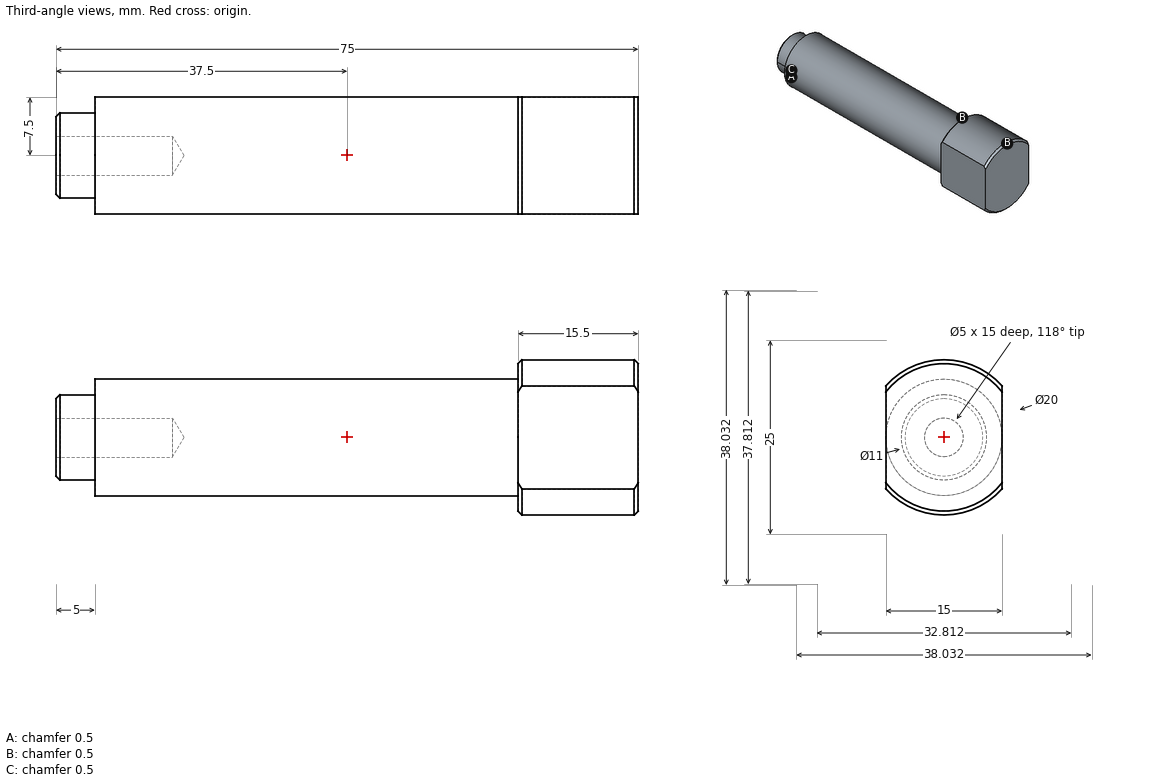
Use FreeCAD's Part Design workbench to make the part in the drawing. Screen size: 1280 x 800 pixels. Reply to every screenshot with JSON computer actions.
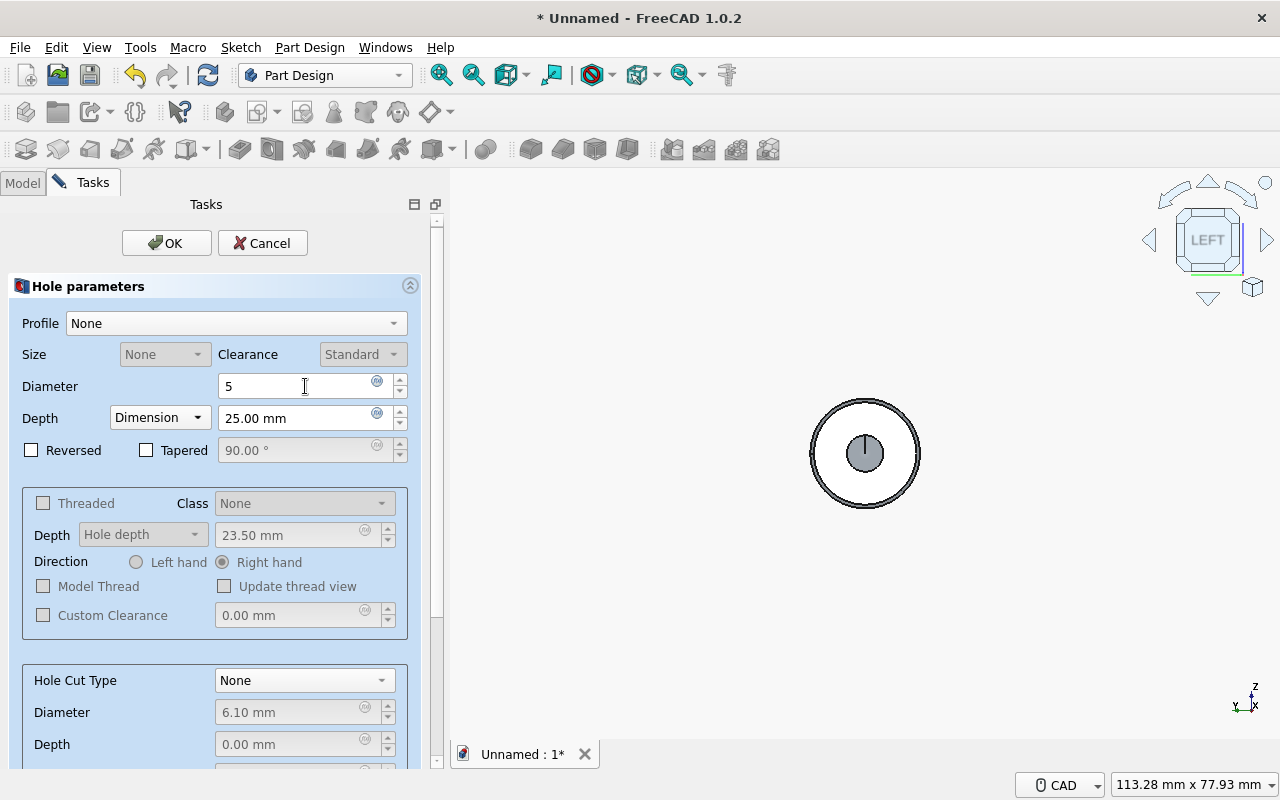
{"action": "triple_click", "coordinate": [305, 418]}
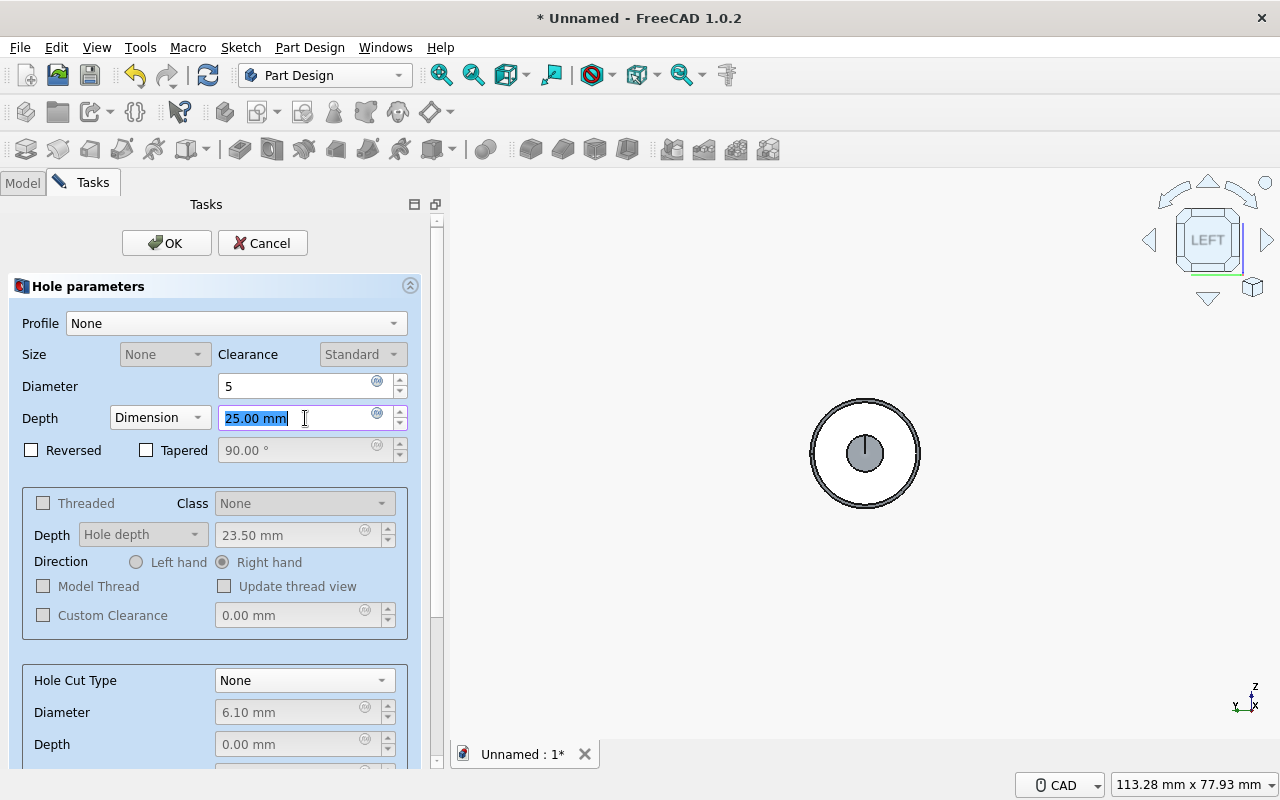
{"action": "type", "text": "15"}
{"action": "key", "text": "Tab"}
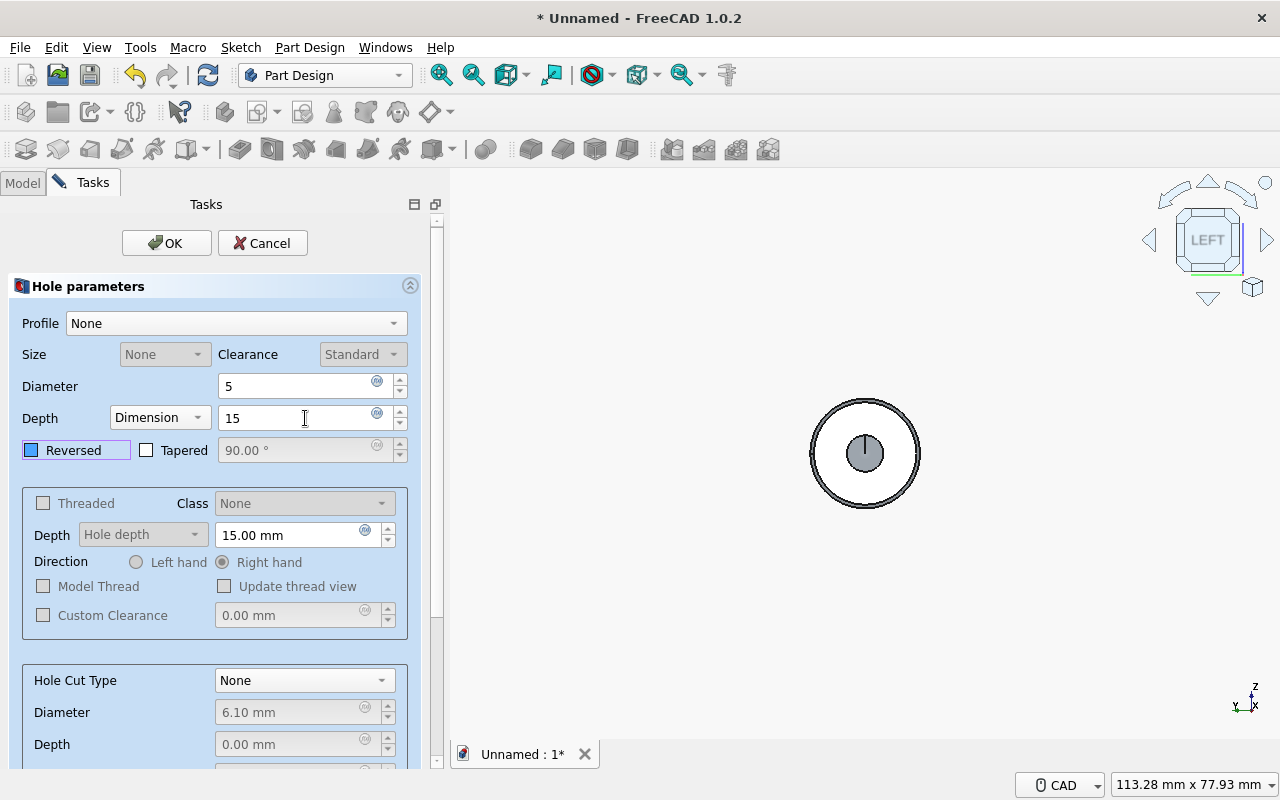
{"action": "left_click", "coordinate": [167, 243]}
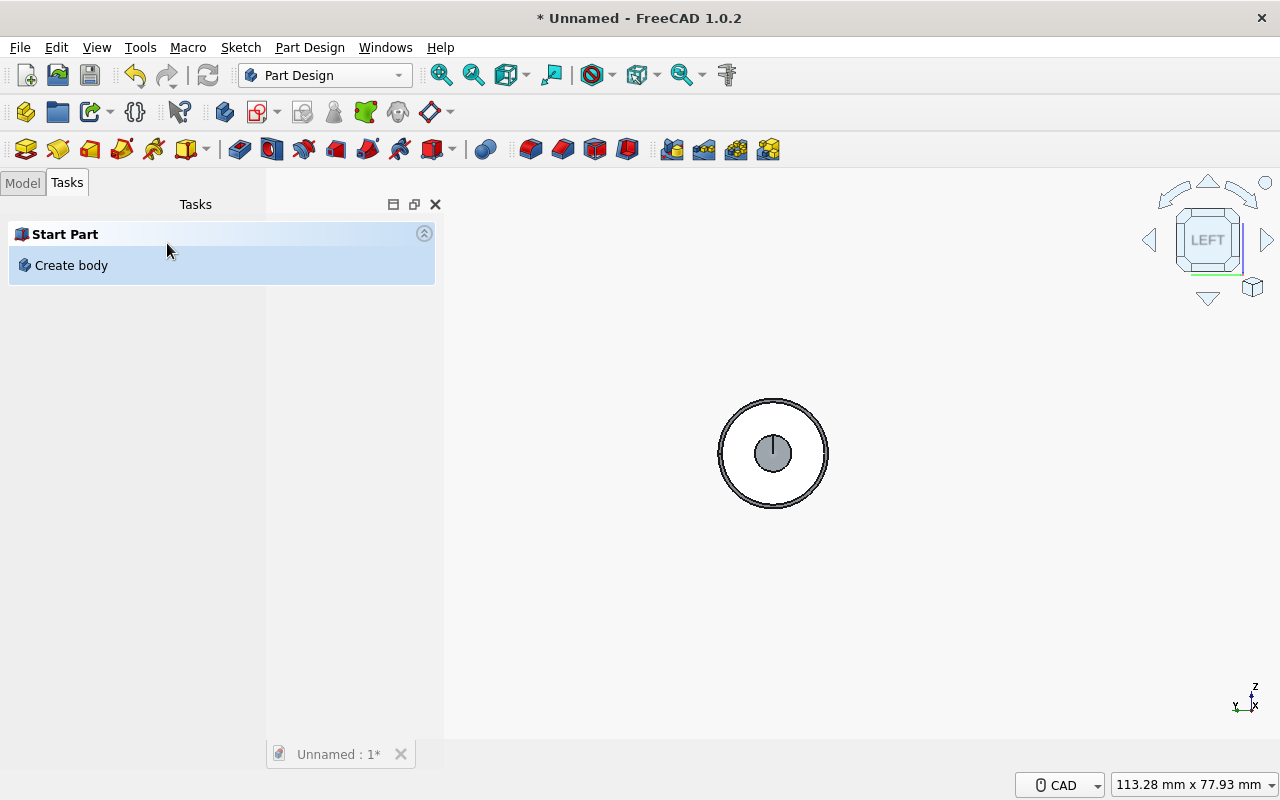
{"action": "key", "text": "v f"}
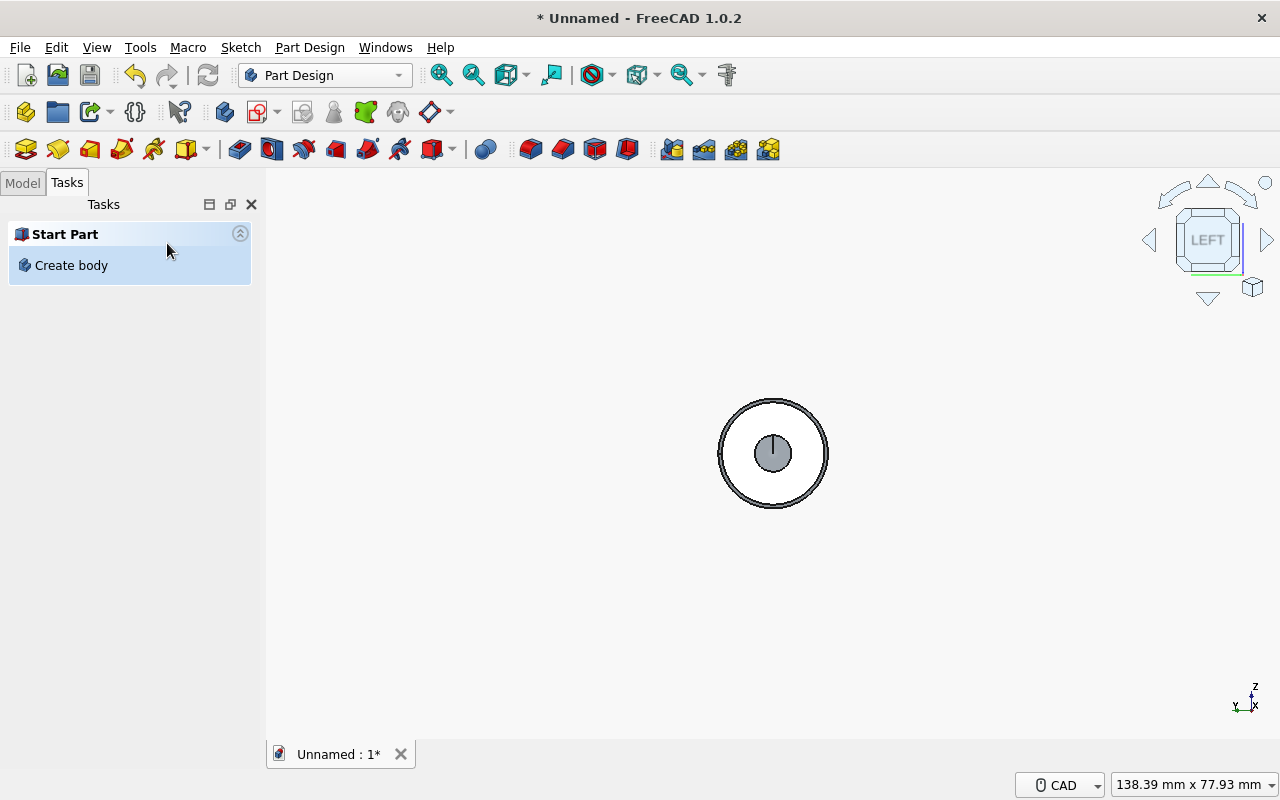
{"action": "key", "text": "0"}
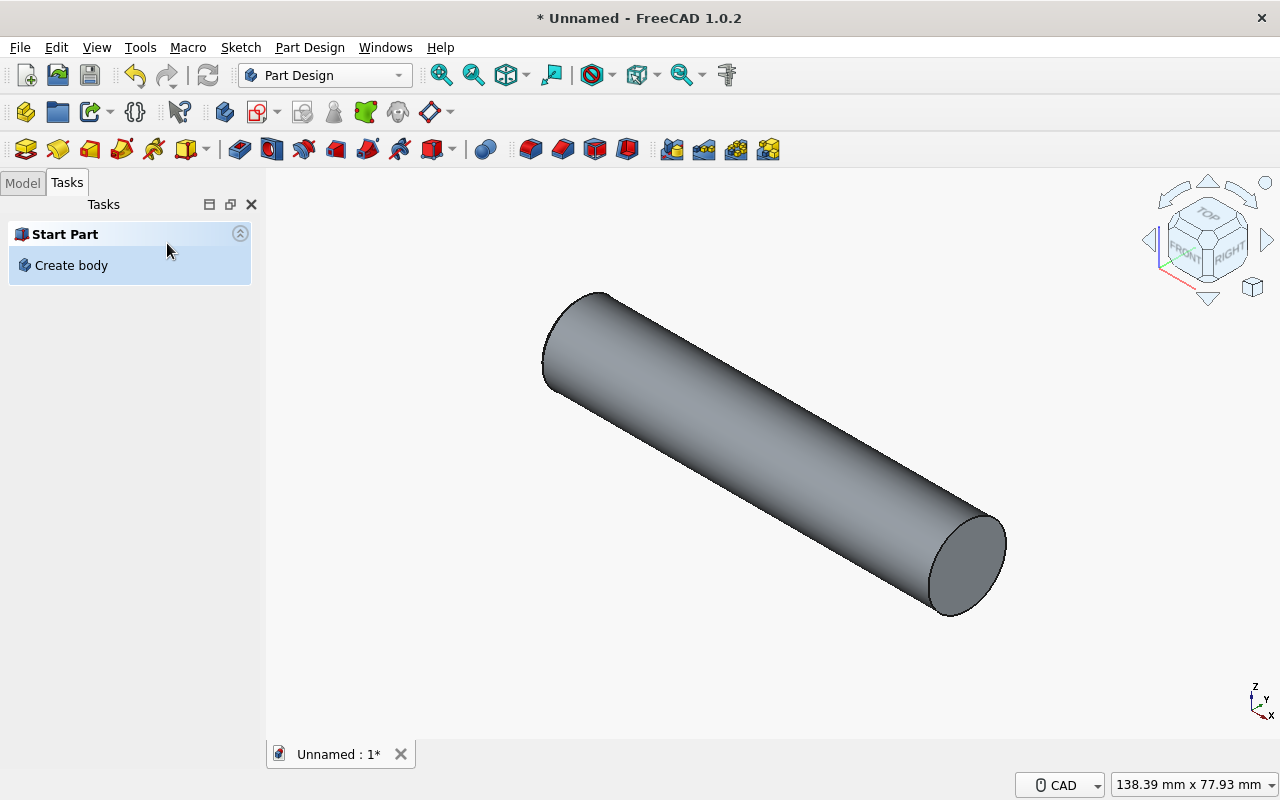
{"action": "left_click", "coordinate": [967, 565]}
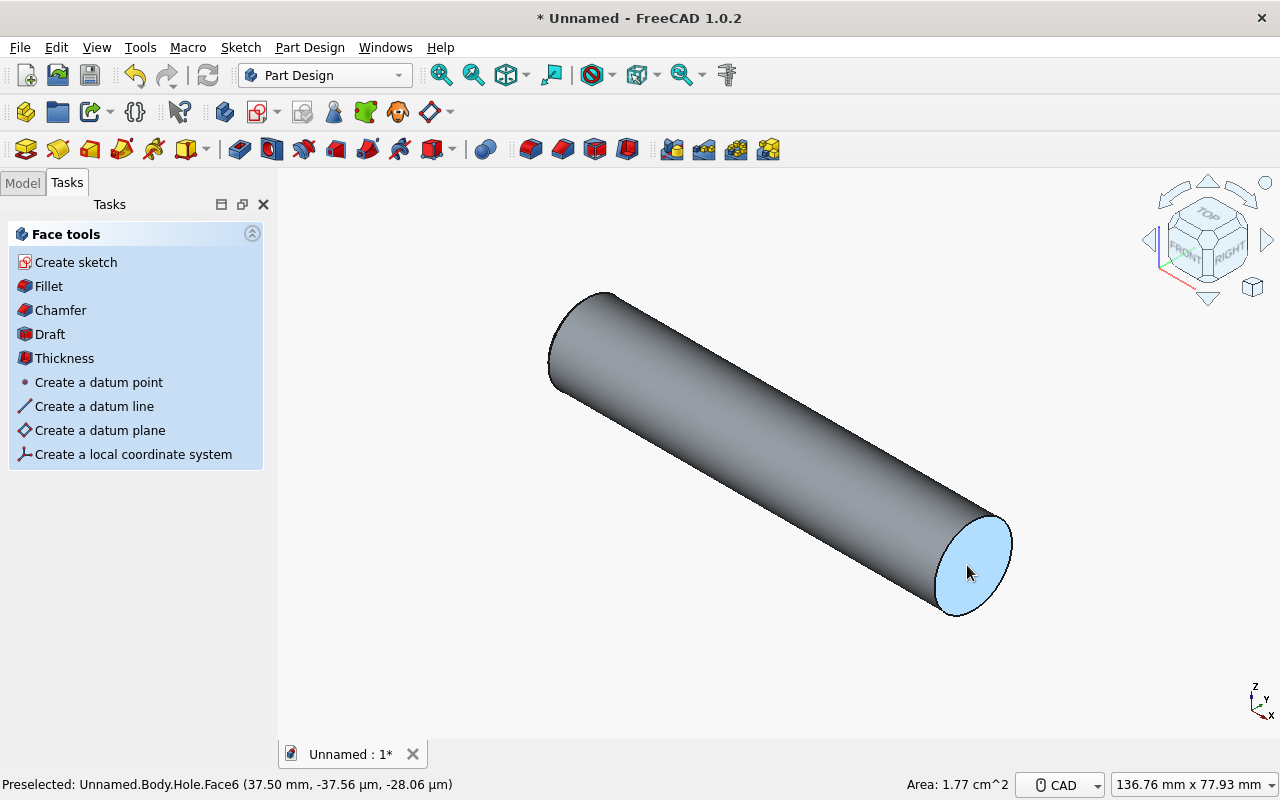
{"action": "left_click", "coordinate": [258, 112]}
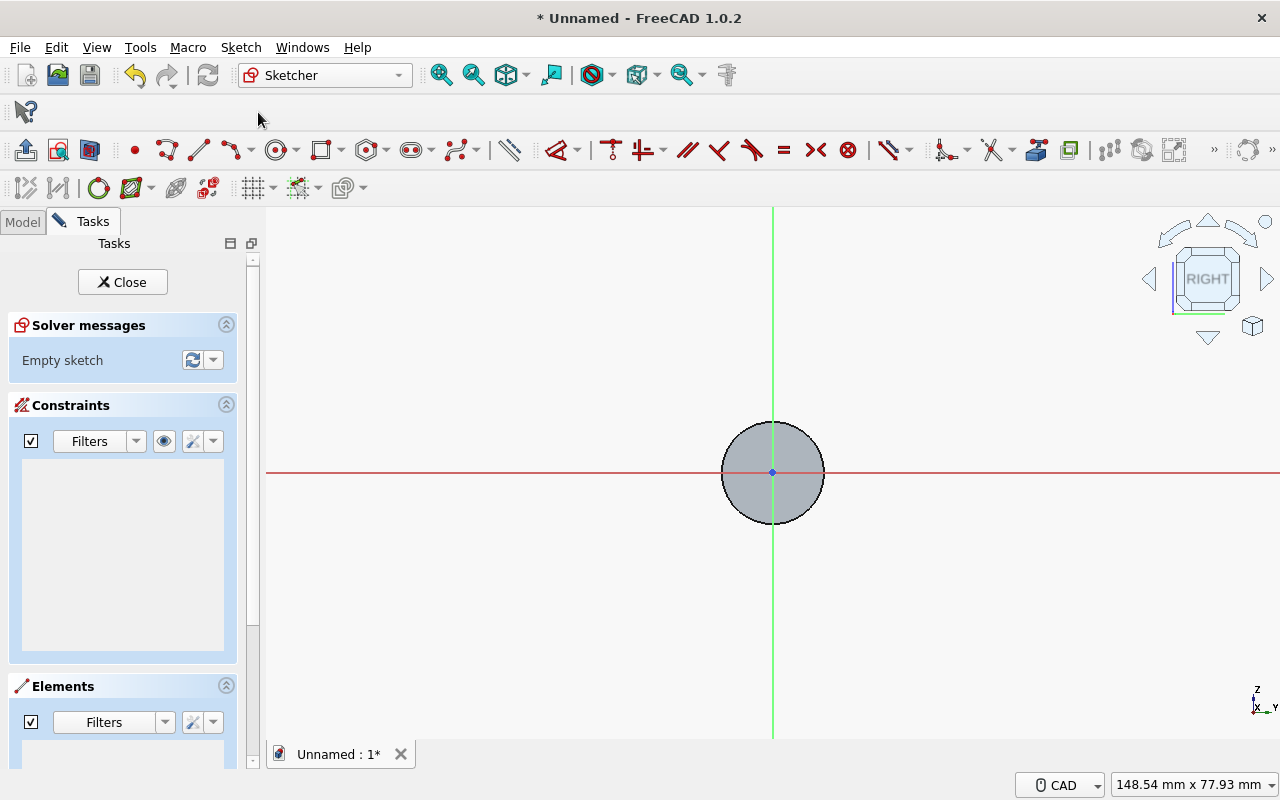
{"action": "scroll", "coordinate": [813, 473], "scroll_direction": "up", "scroll_amount": 5}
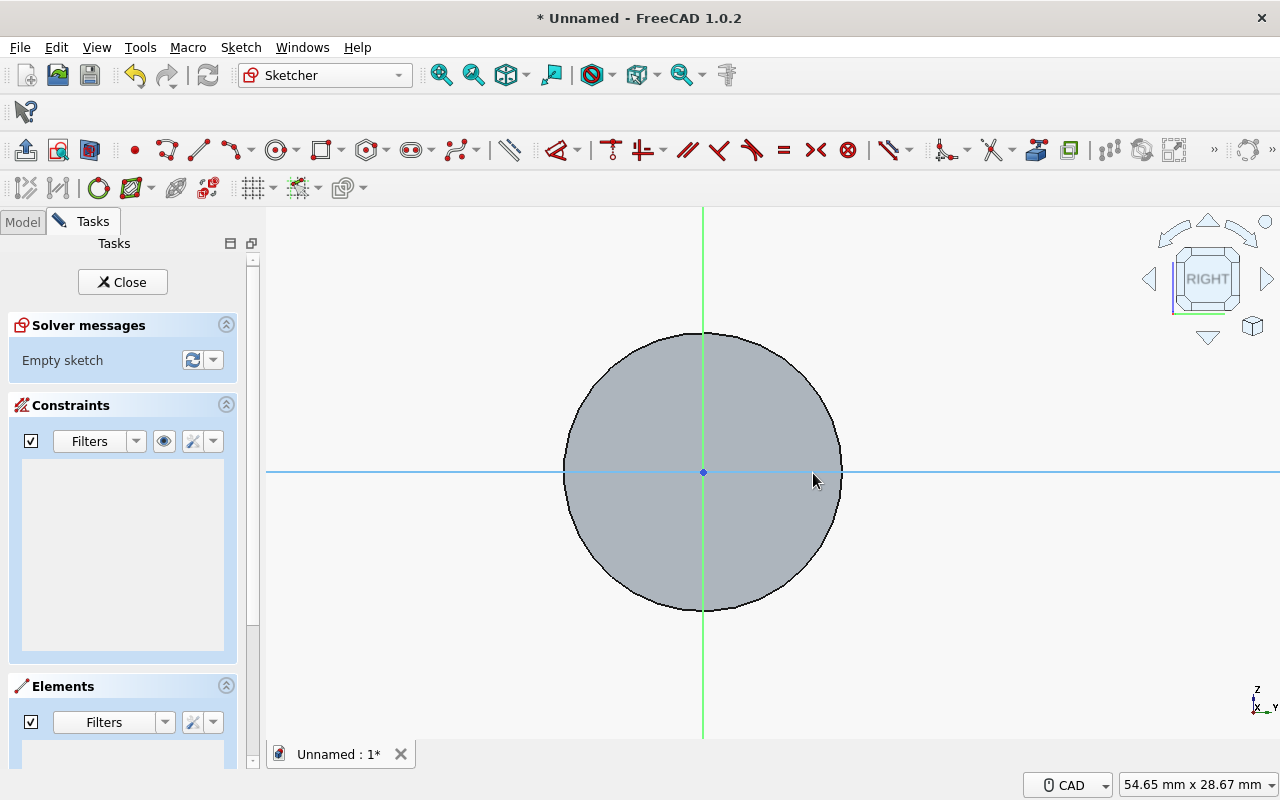
{"action": "left_click", "coordinate": [276, 150]}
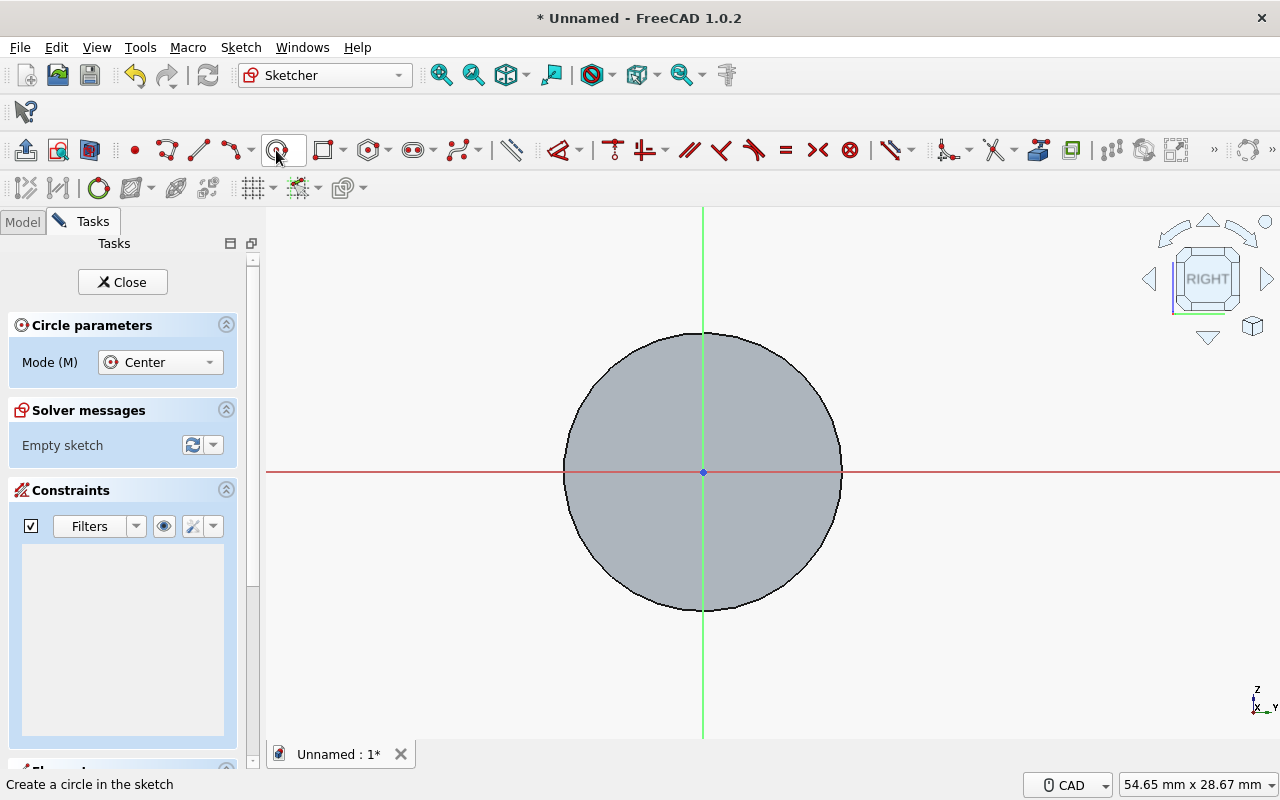
{"action": "left_click", "coordinate": [703, 472]}
{"action": "left_click", "coordinate": [834, 341]}
{"action": "key", "text": "Escape"}